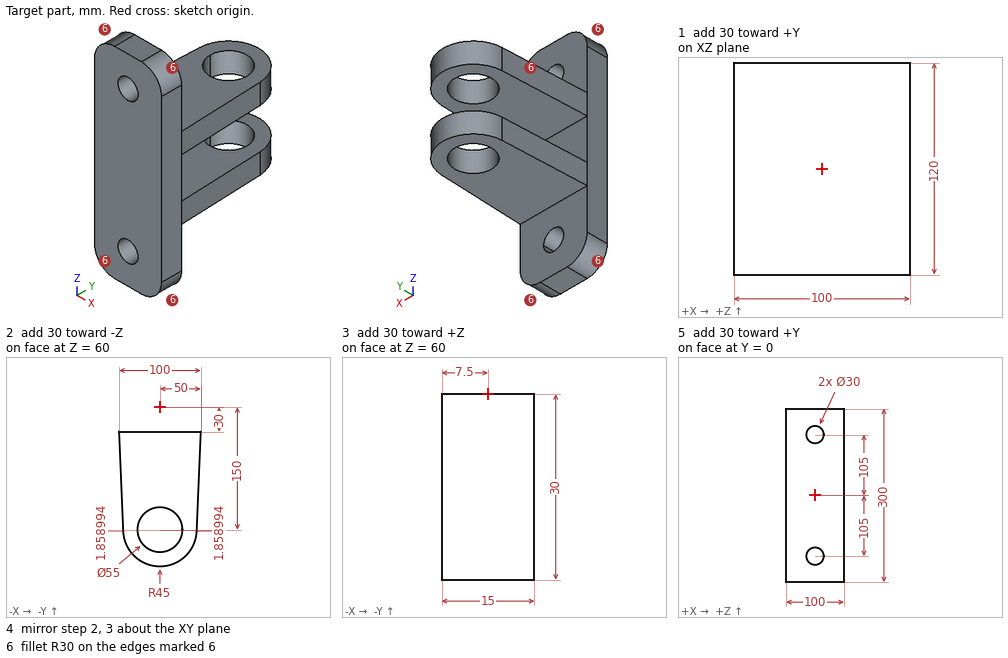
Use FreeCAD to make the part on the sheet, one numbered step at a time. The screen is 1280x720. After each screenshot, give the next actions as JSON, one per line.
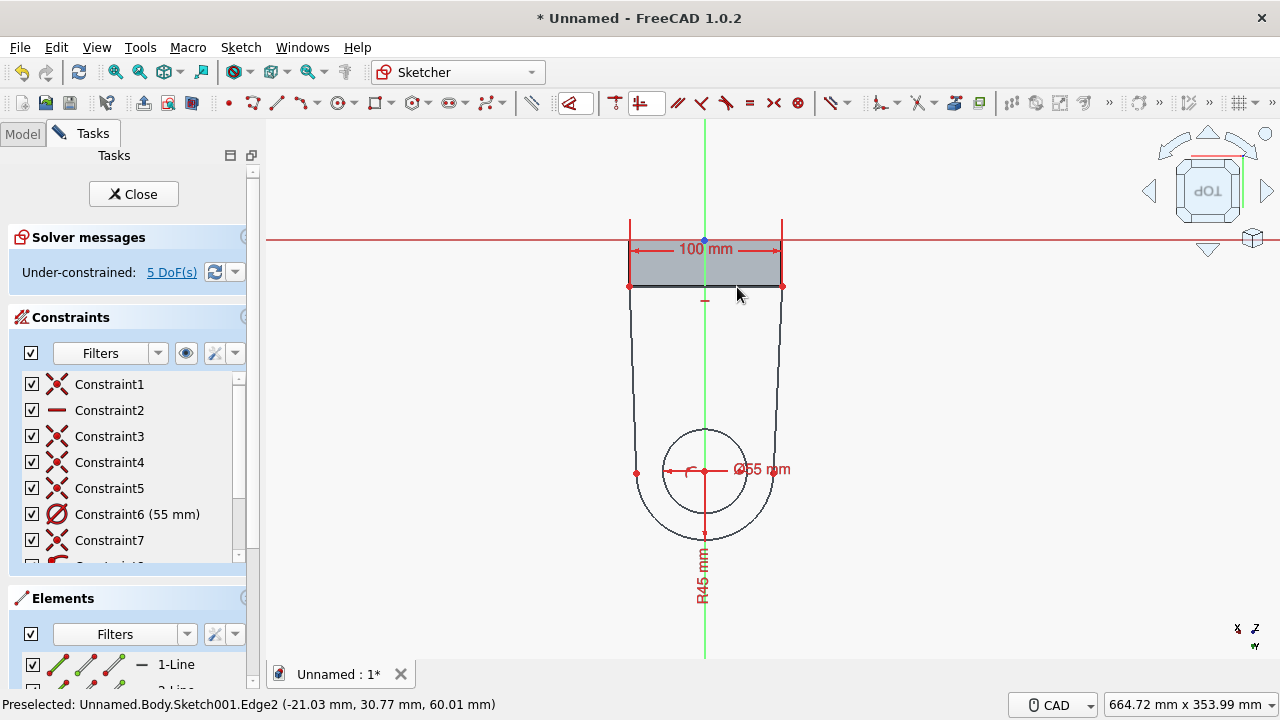
{"action": "left_click", "coordinate": [782, 287]}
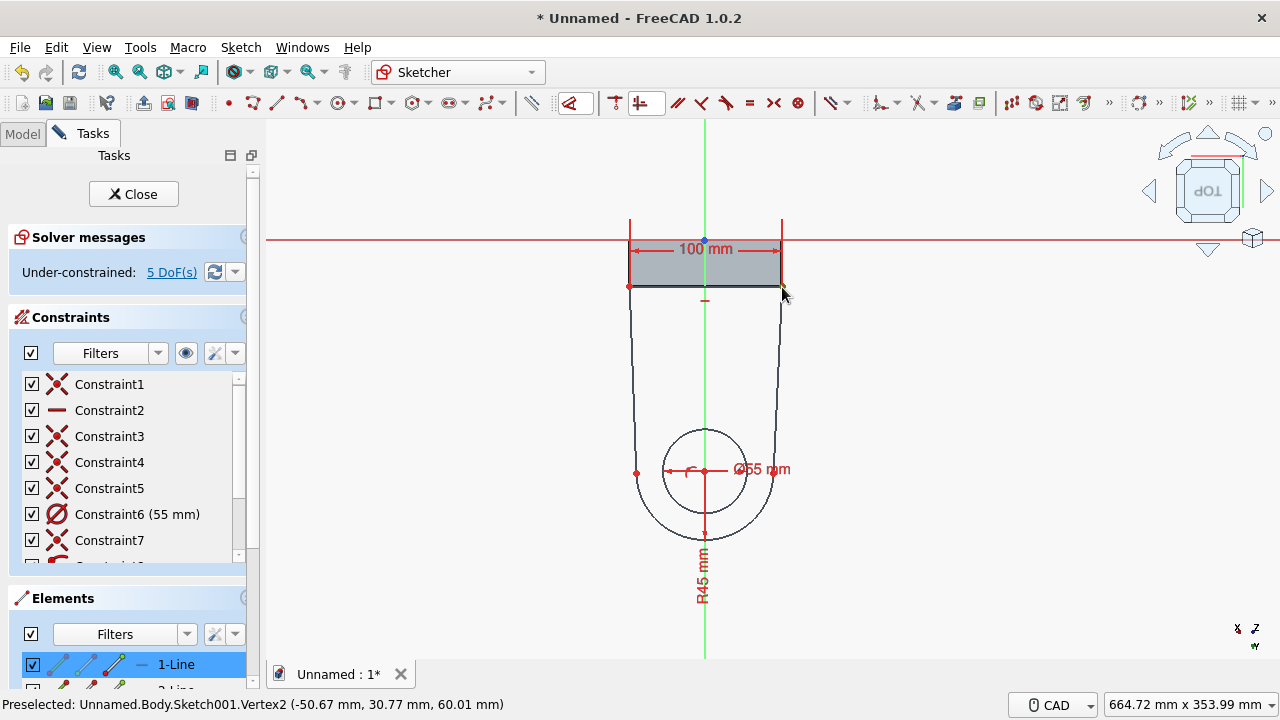
{"action": "key", "text": "l"}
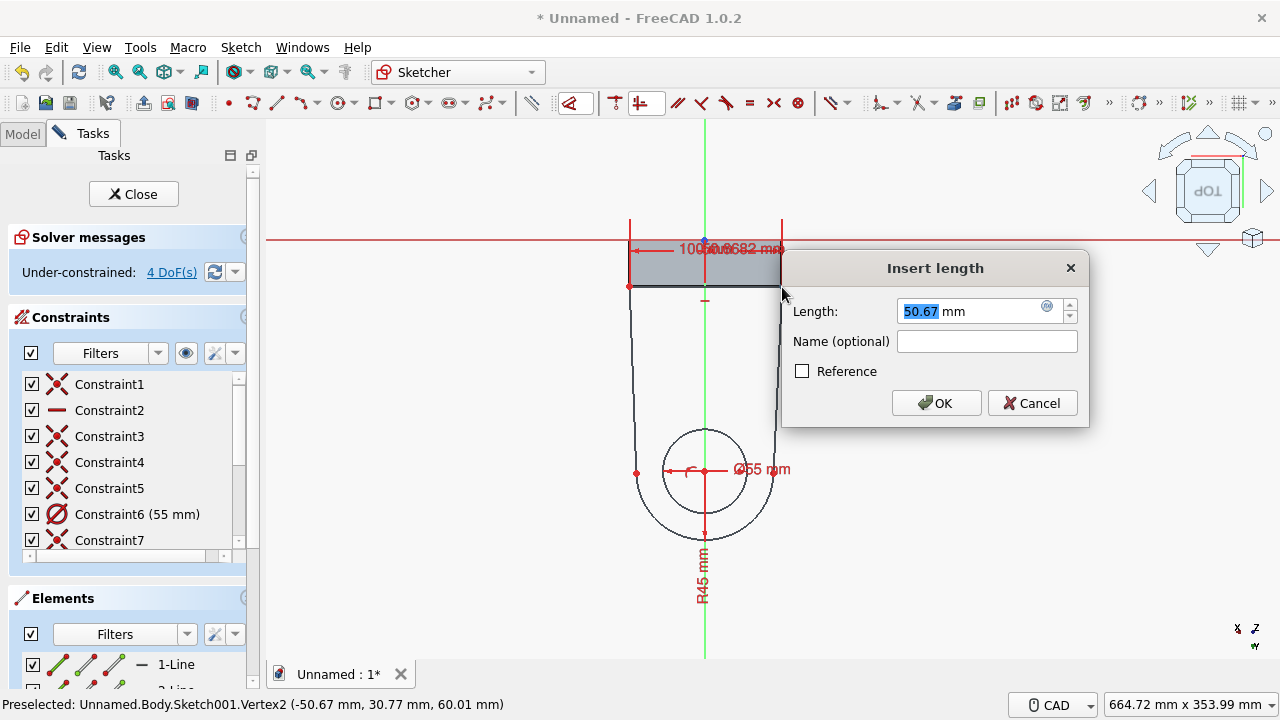
{"action": "type", "text": "50"}
{"action": "key", "text": "Return"}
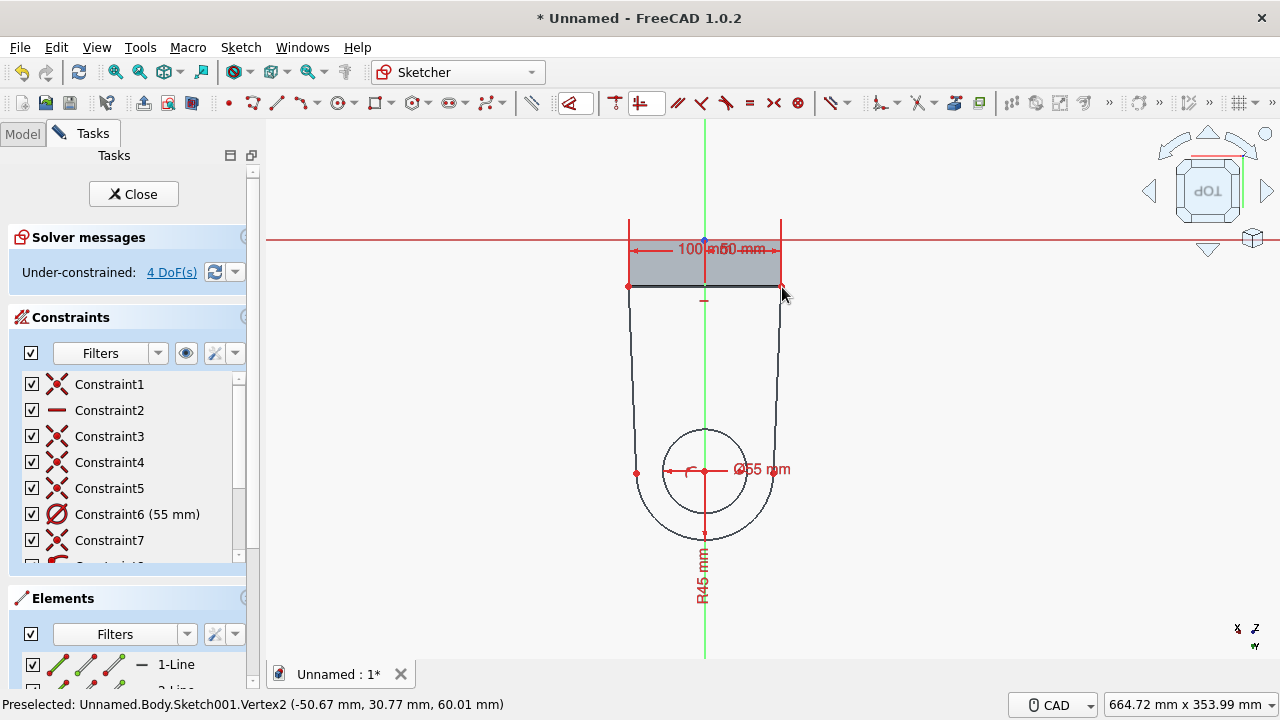
{"action": "left_click", "coordinate": [781, 287]}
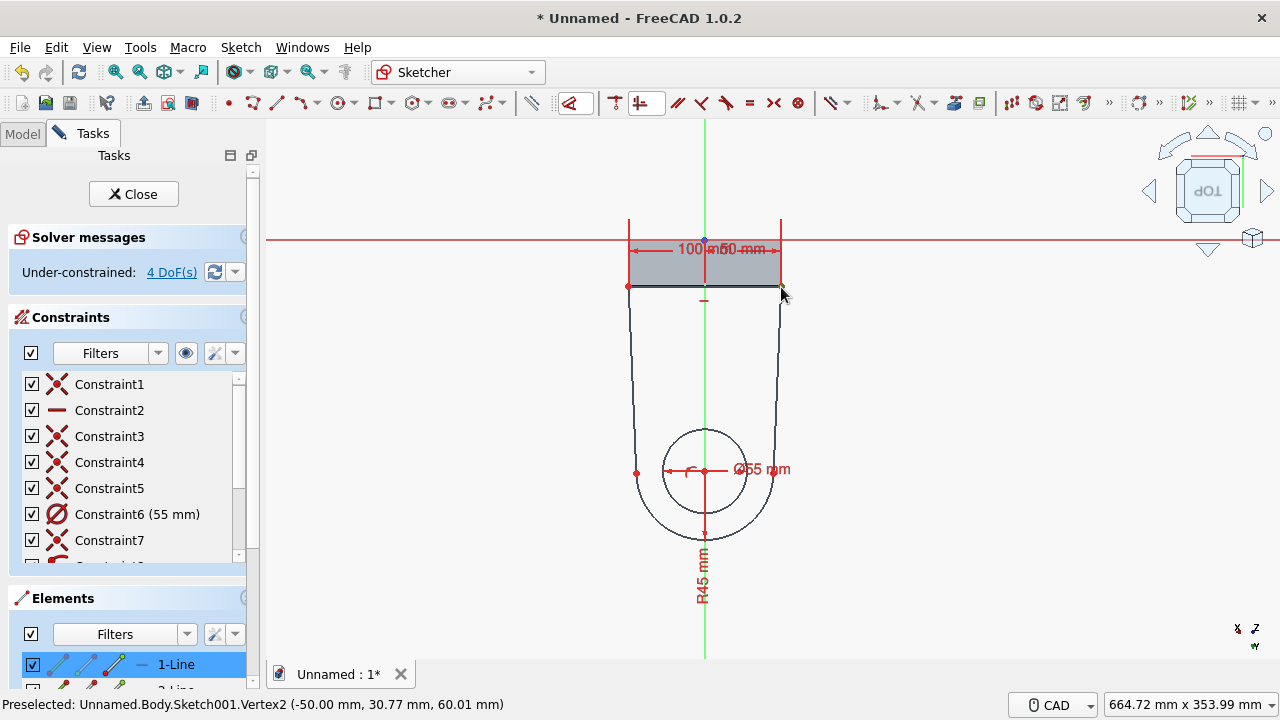
{"action": "key", "text": "i"}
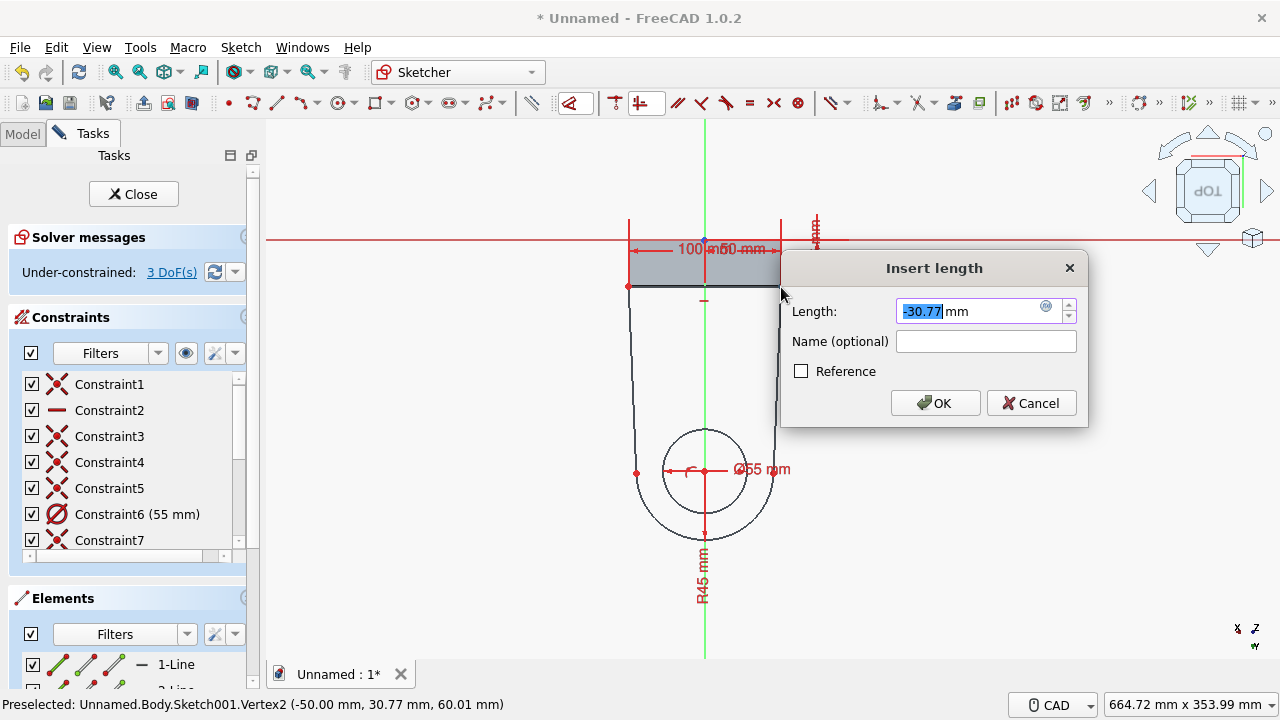
{"action": "type", "text": "-30"}
{"action": "key", "text": "Return"}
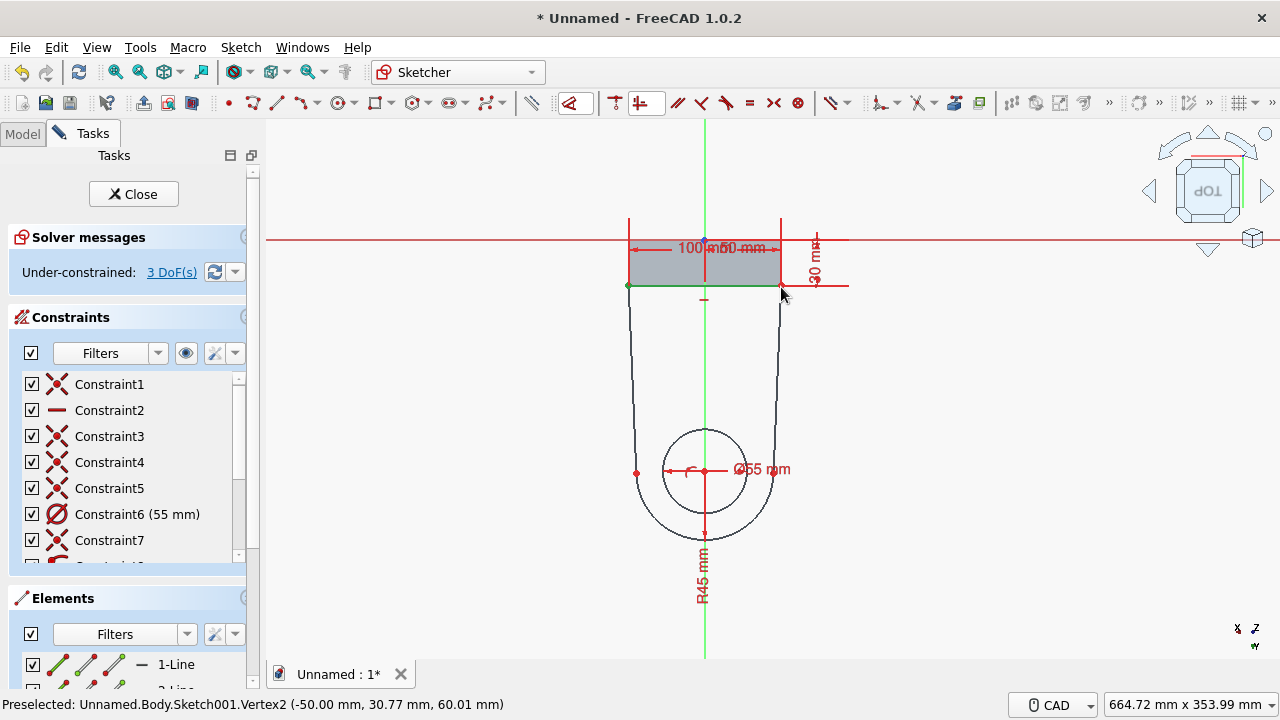
{"action": "left_click", "coordinate": [705, 471]}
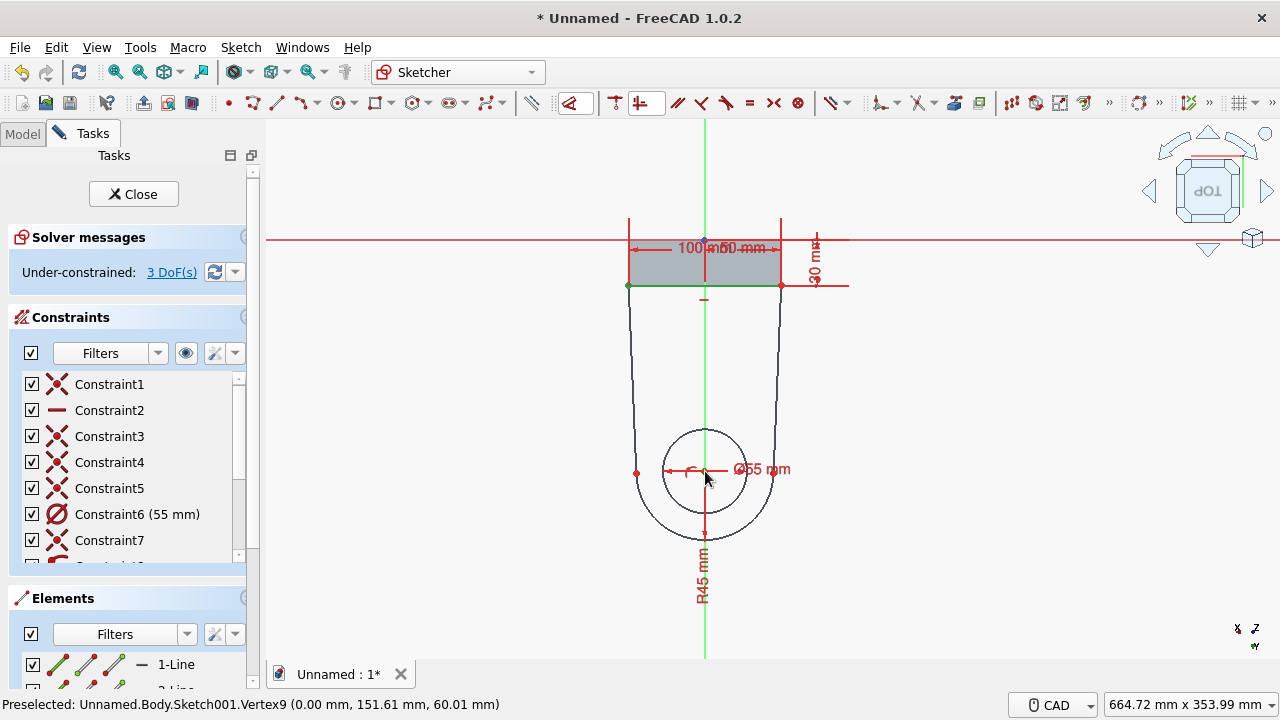
{"action": "key", "text": "i"}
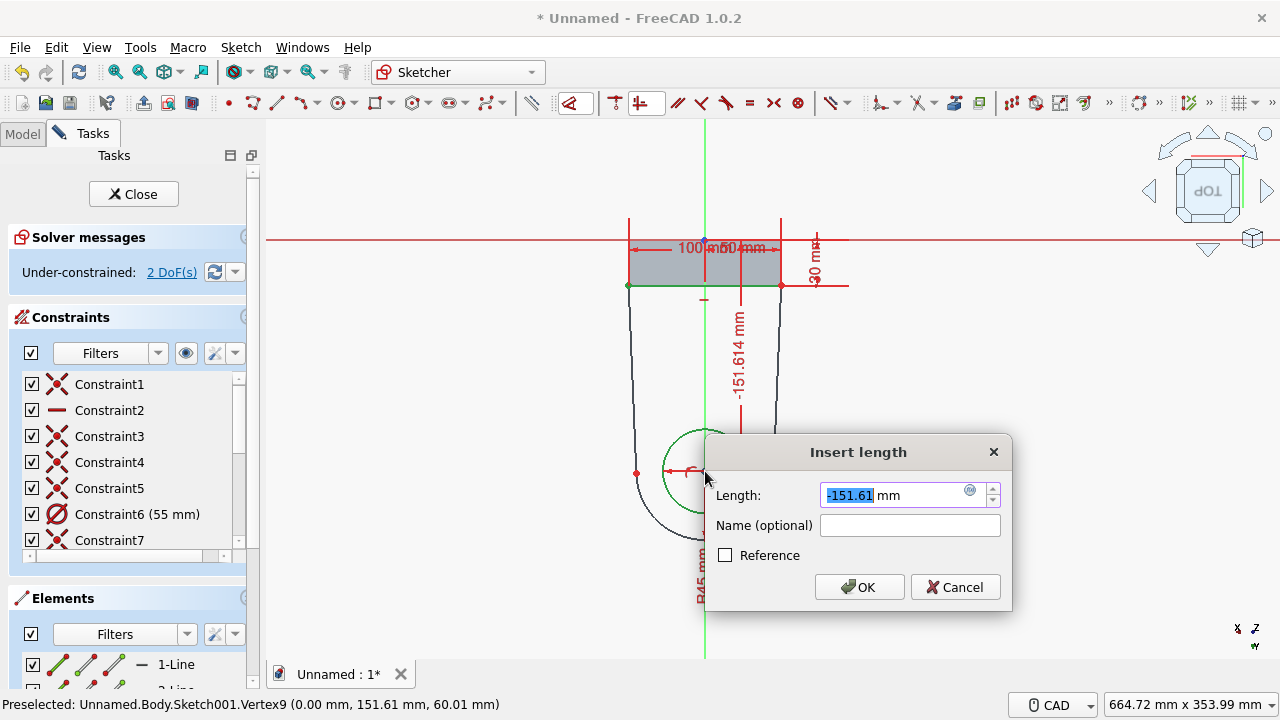
{"action": "type", "text": "-150"}
{"action": "key", "text": "Return"}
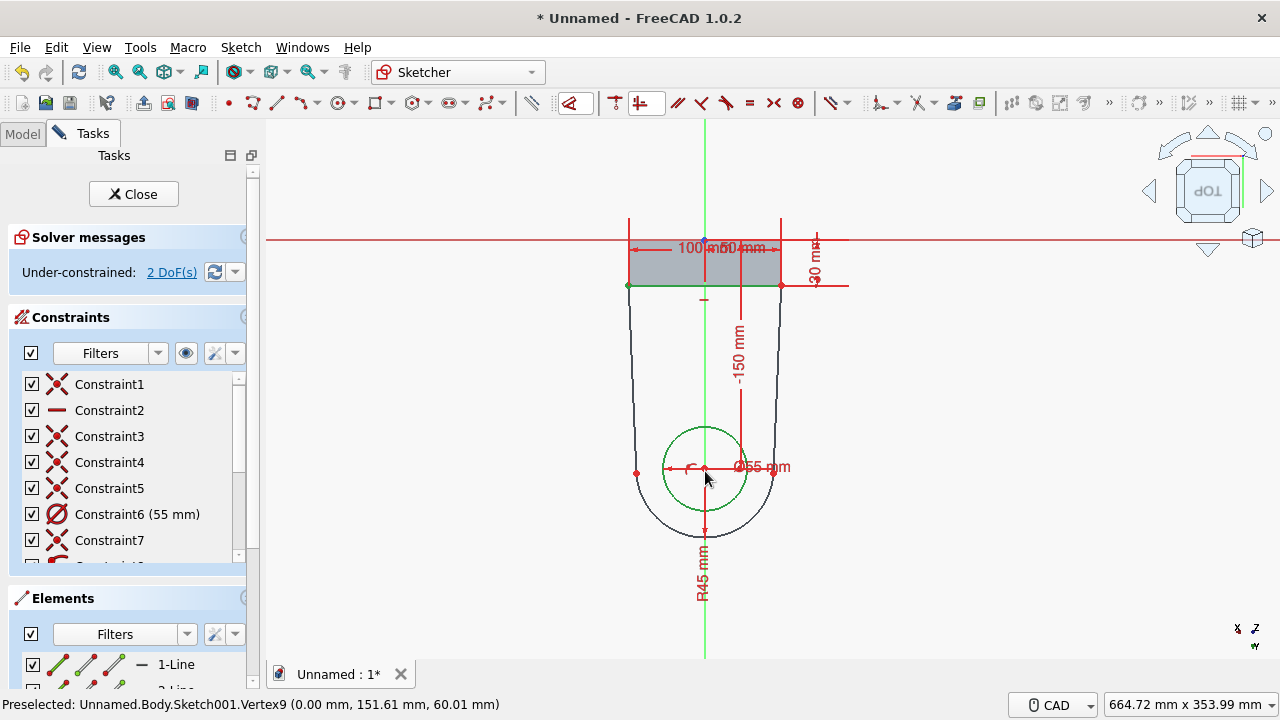
{"action": "scroll", "coordinate": [636, 473], "scroll_direction": "up", "scroll_amount": 14}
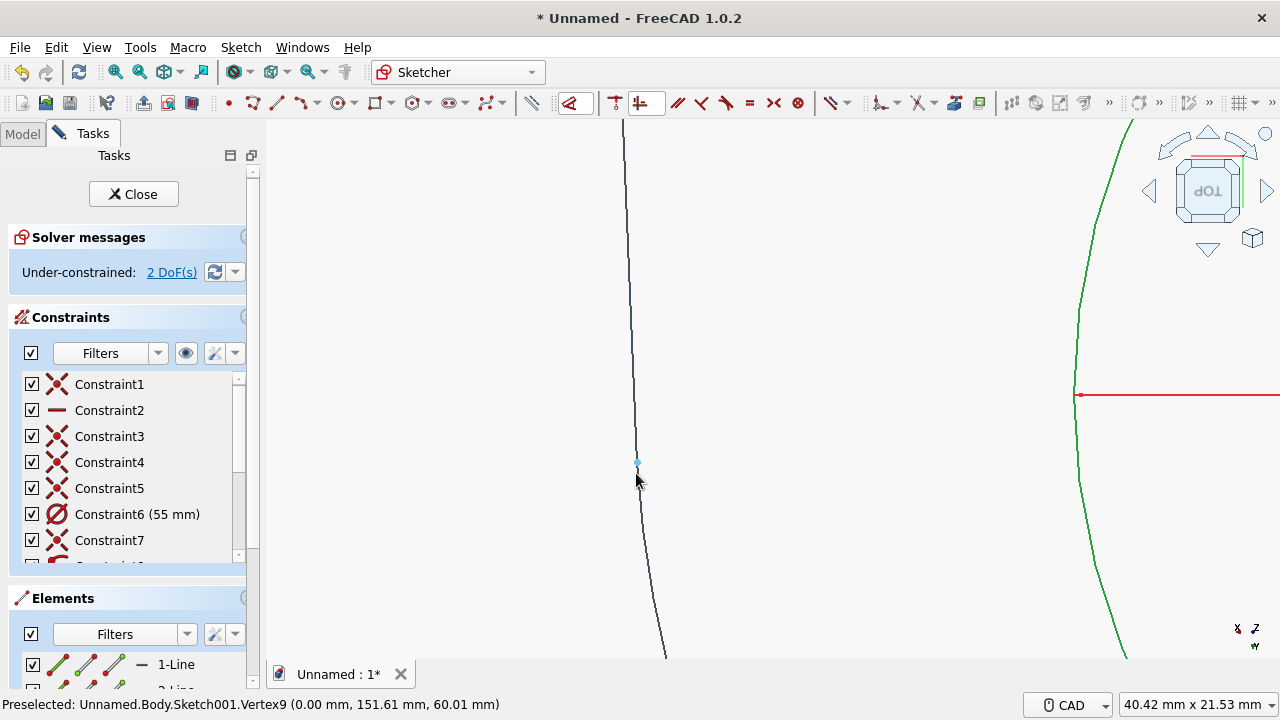
{"action": "left_click", "coordinate": [637, 463]}